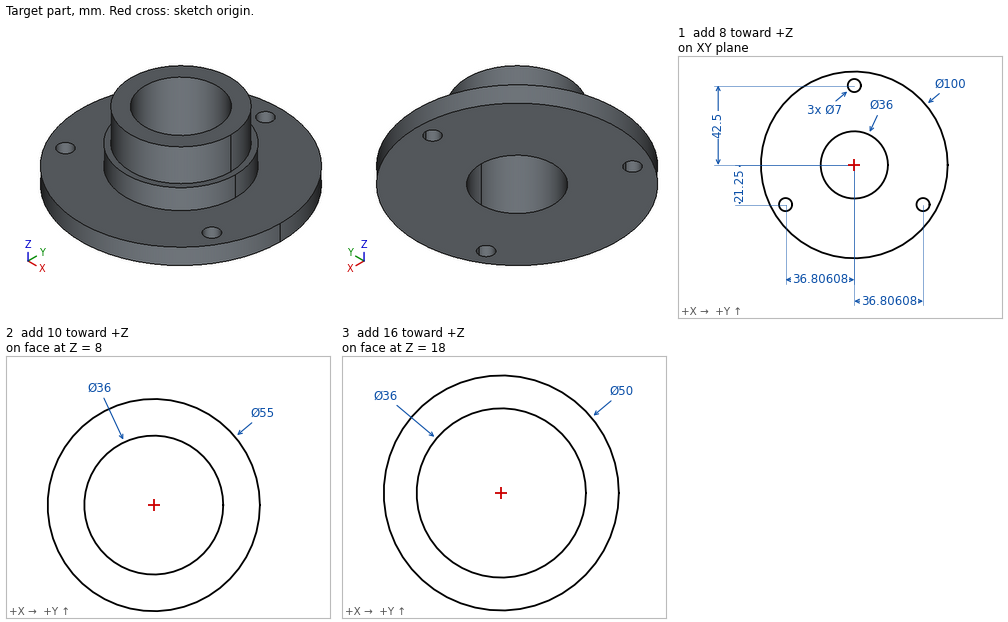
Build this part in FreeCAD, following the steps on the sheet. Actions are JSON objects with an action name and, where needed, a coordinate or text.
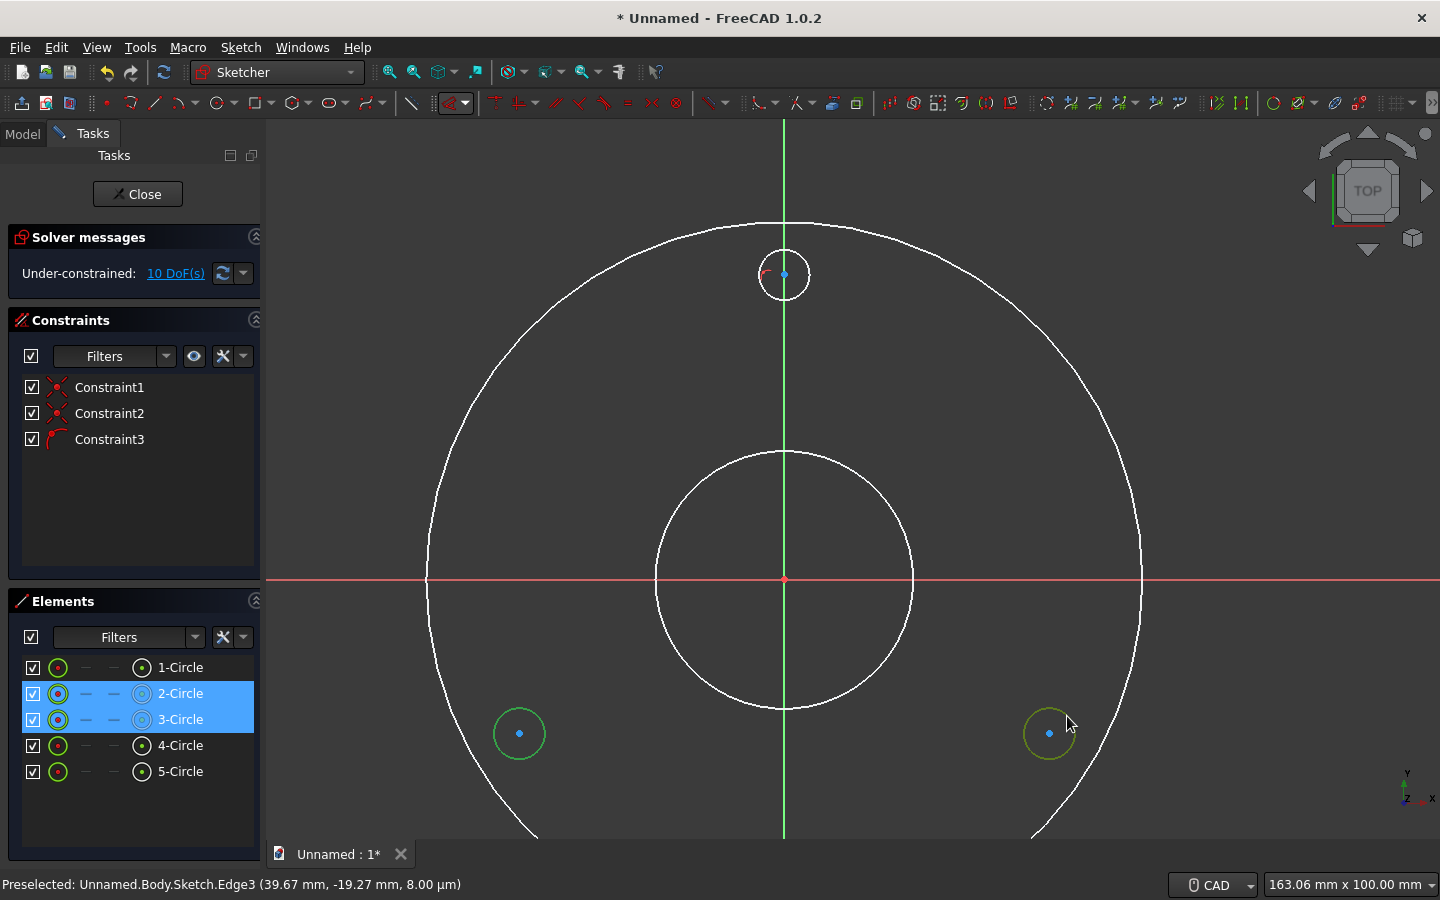
{"action": "left_click", "coordinate": [802, 257]}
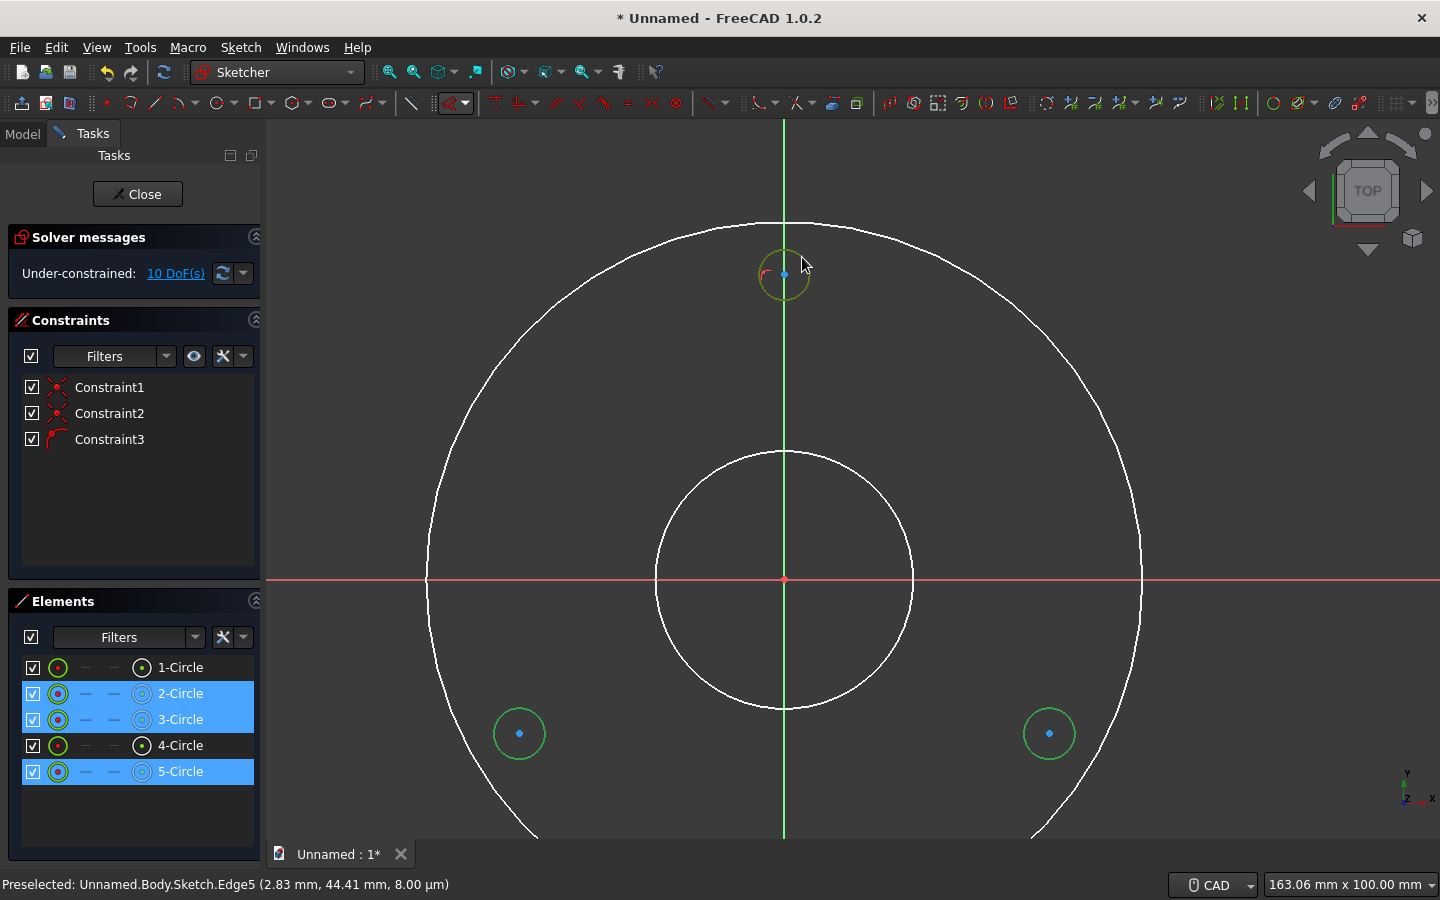
{"action": "left_click", "coordinate": [628, 104]}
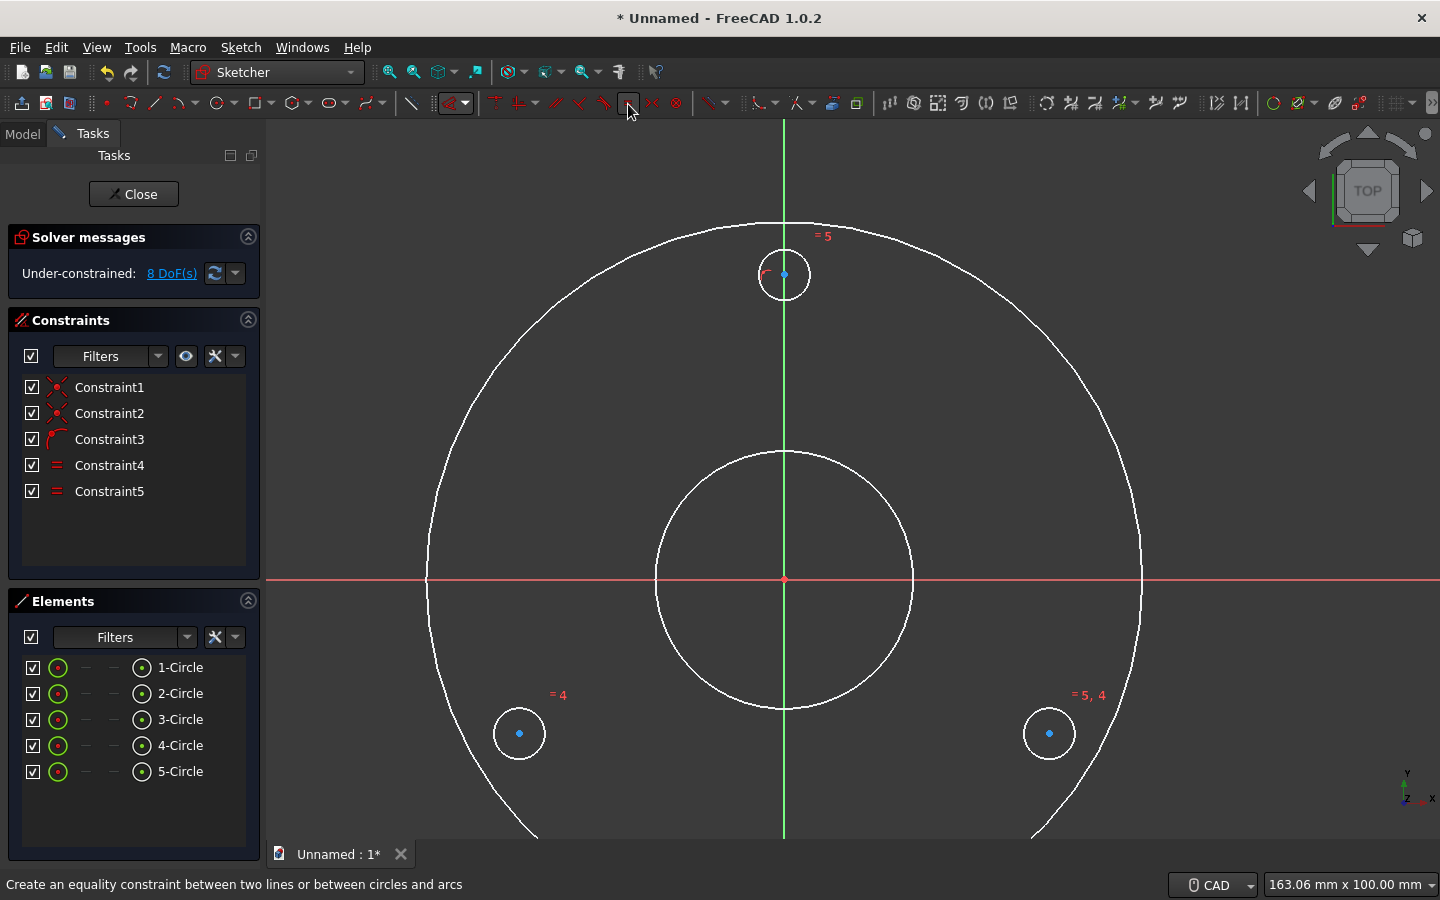
{"action": "left_click", "coordinate": [519, 734]}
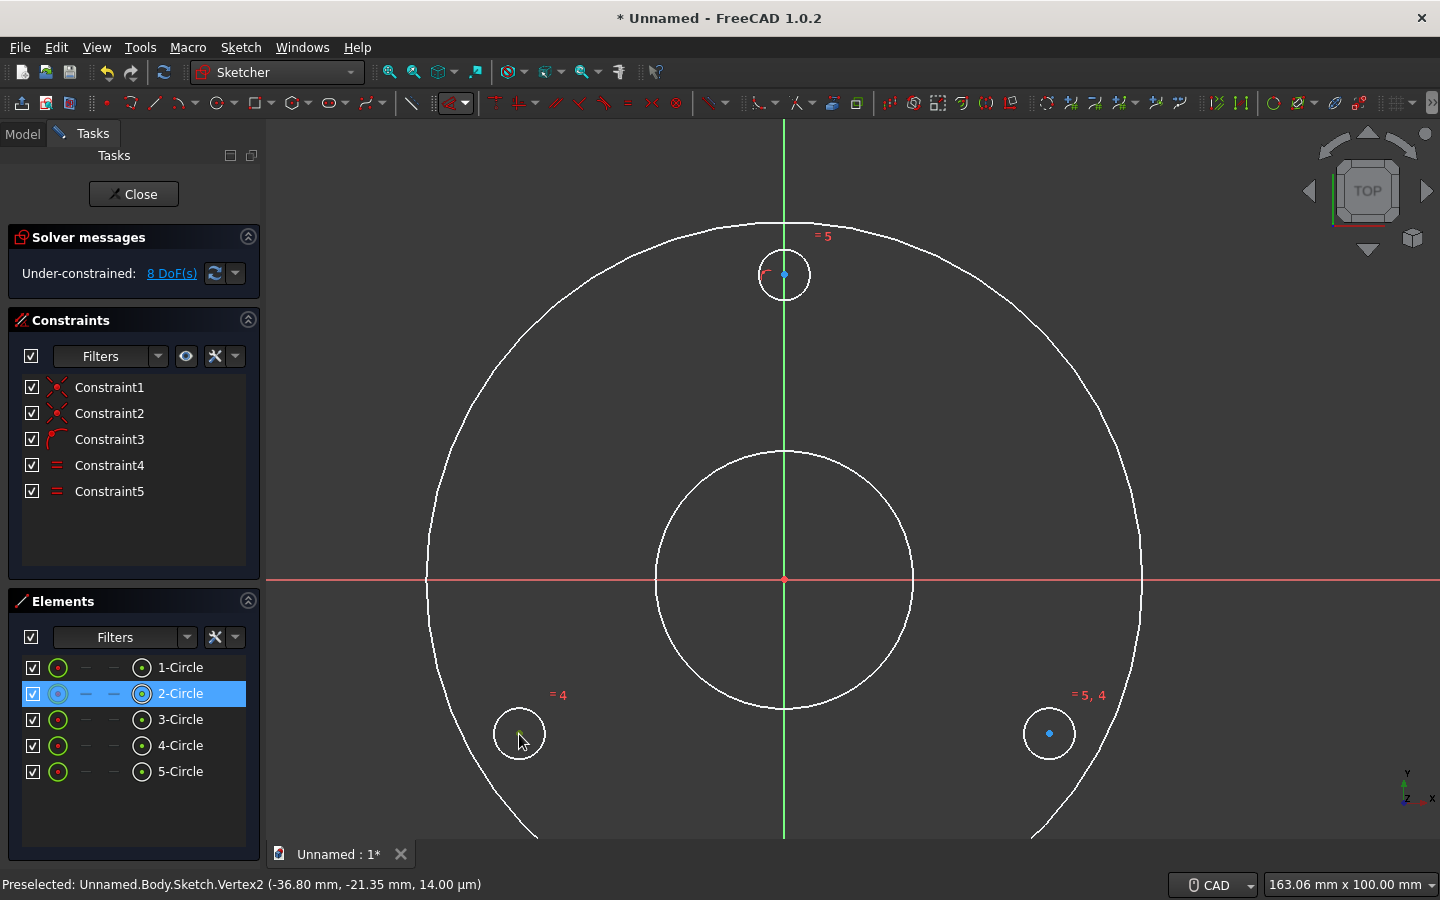
{"action": "left_click", "coordinate": [1049, 734]}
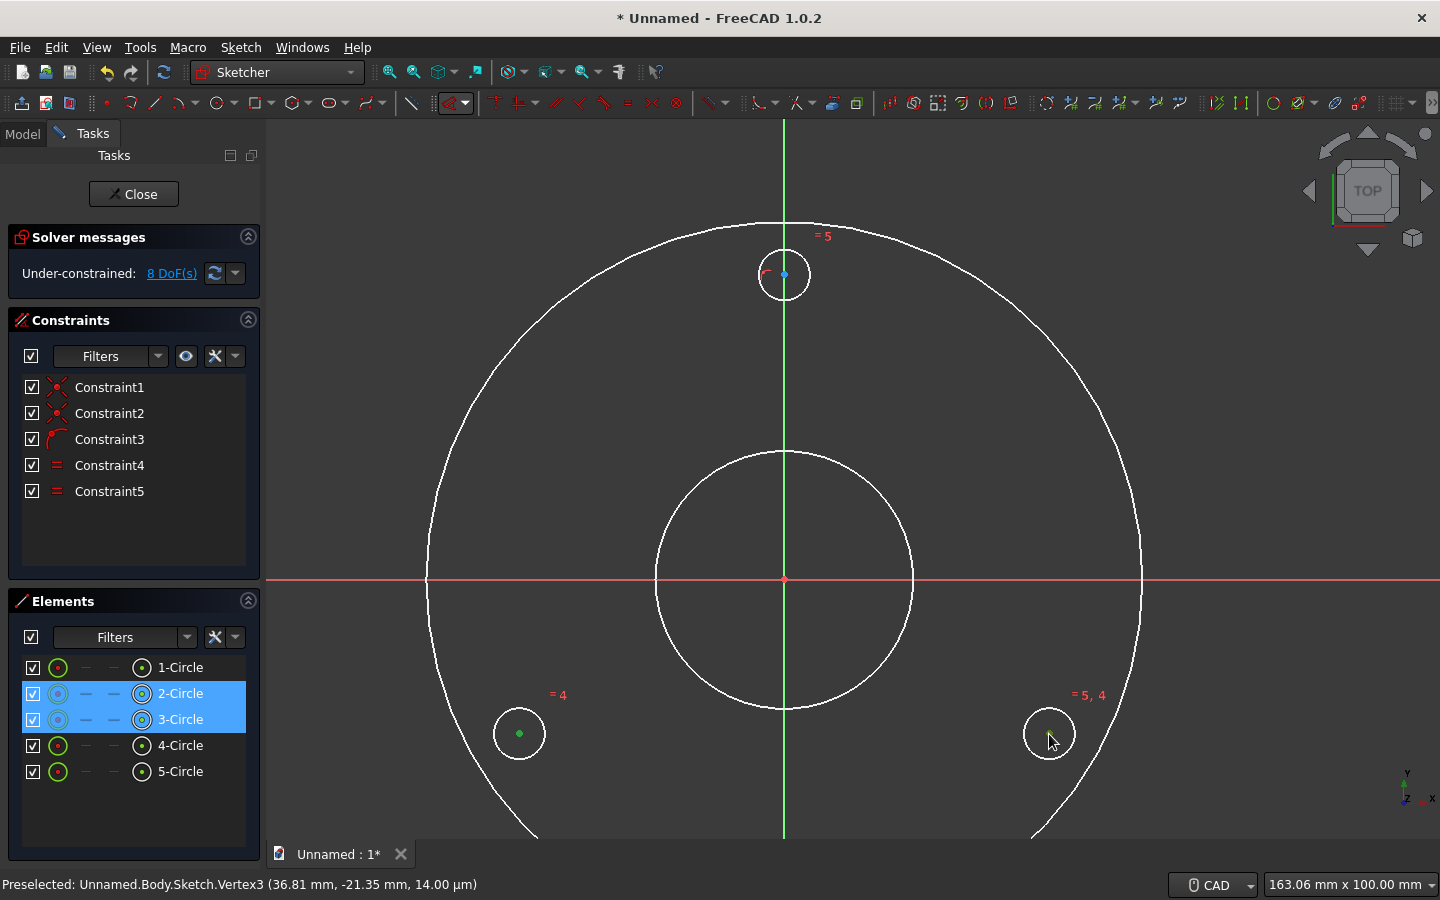
{"action": "left_click", "coordinate": [538, 104]}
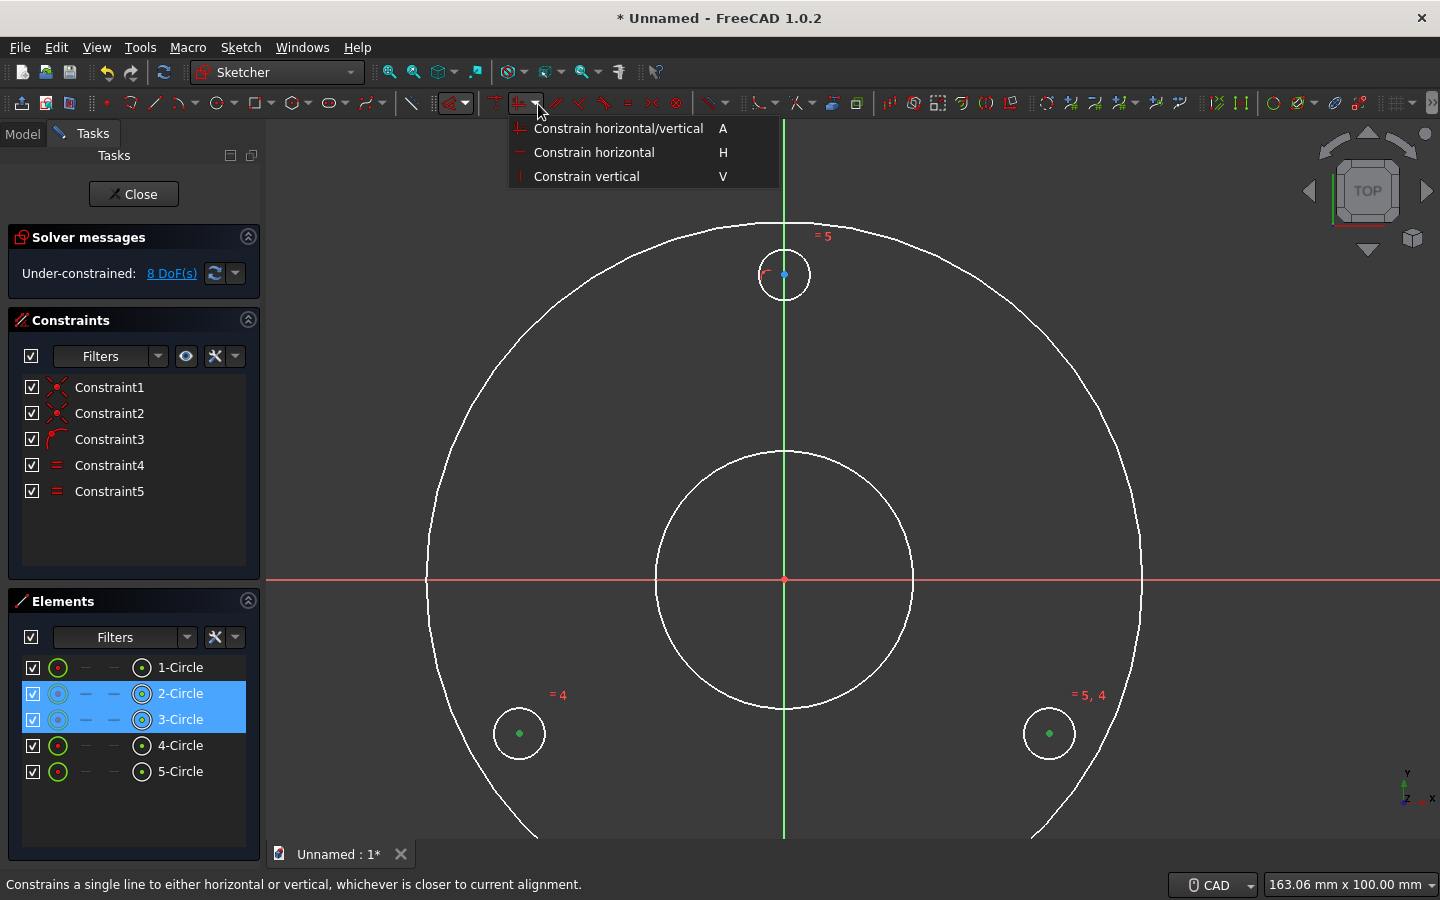
{"action": "left_click", "coordinate": [644, 152]}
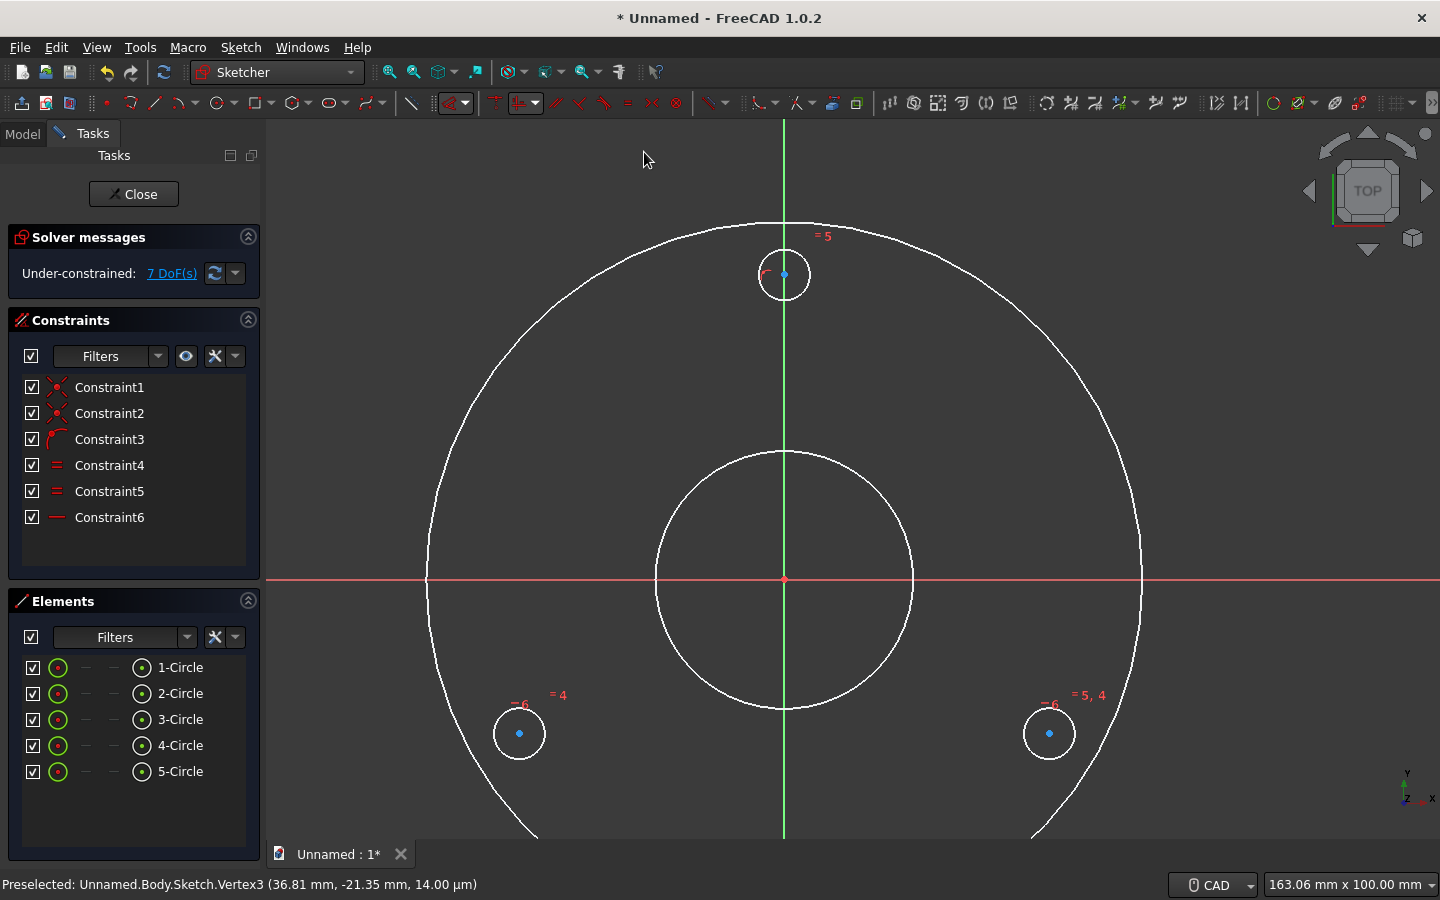
{"action": "left_click", "coordinate": [450, 104]}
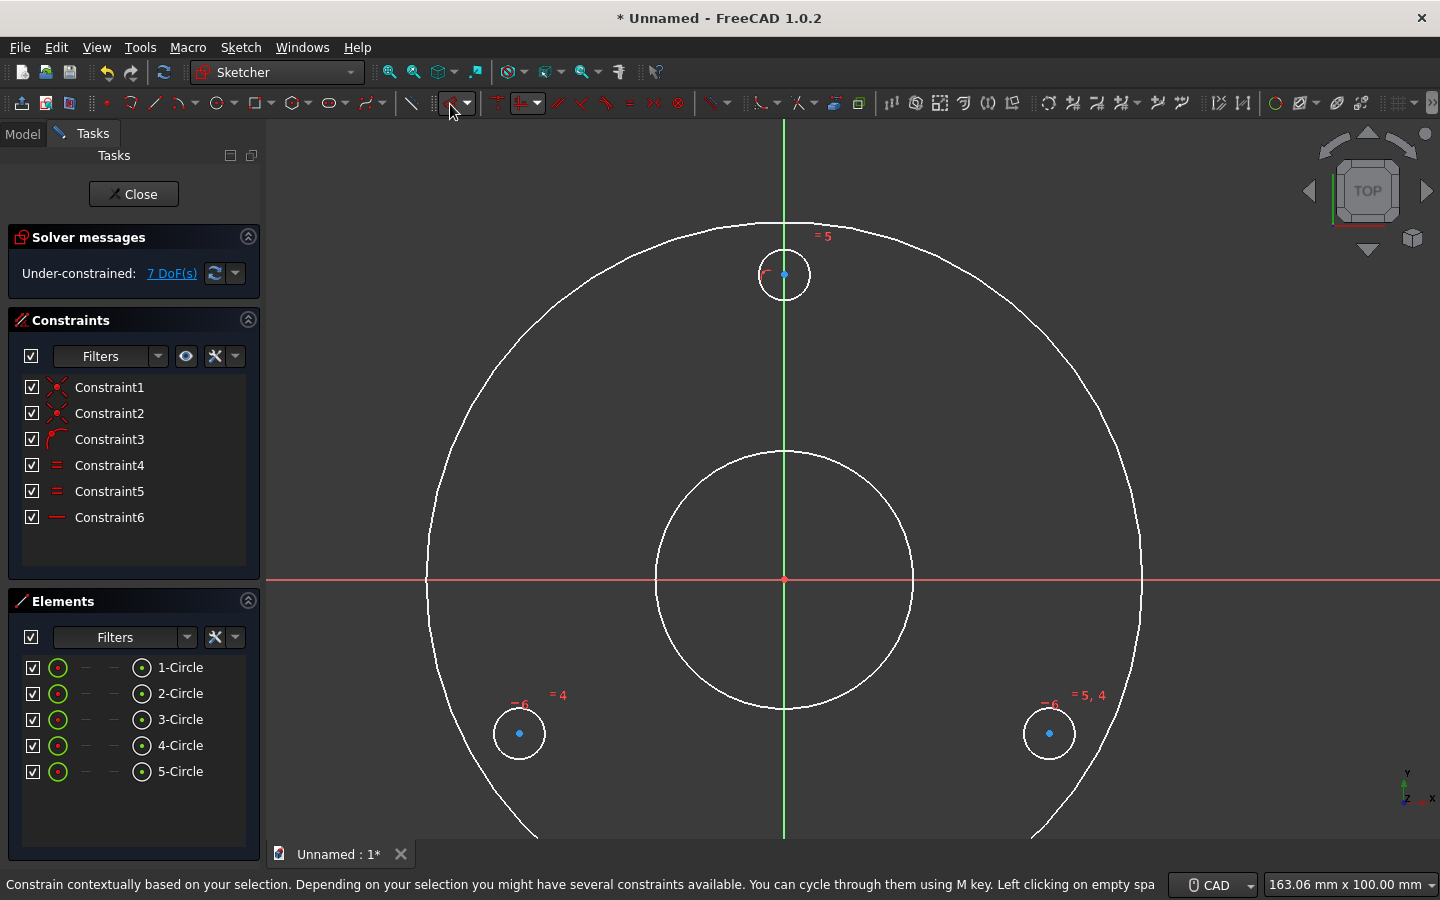
{"action": "left_click", "coordinate": [1037, 326]}
{"action": "left_click", "coordinate": [1060, 303]}